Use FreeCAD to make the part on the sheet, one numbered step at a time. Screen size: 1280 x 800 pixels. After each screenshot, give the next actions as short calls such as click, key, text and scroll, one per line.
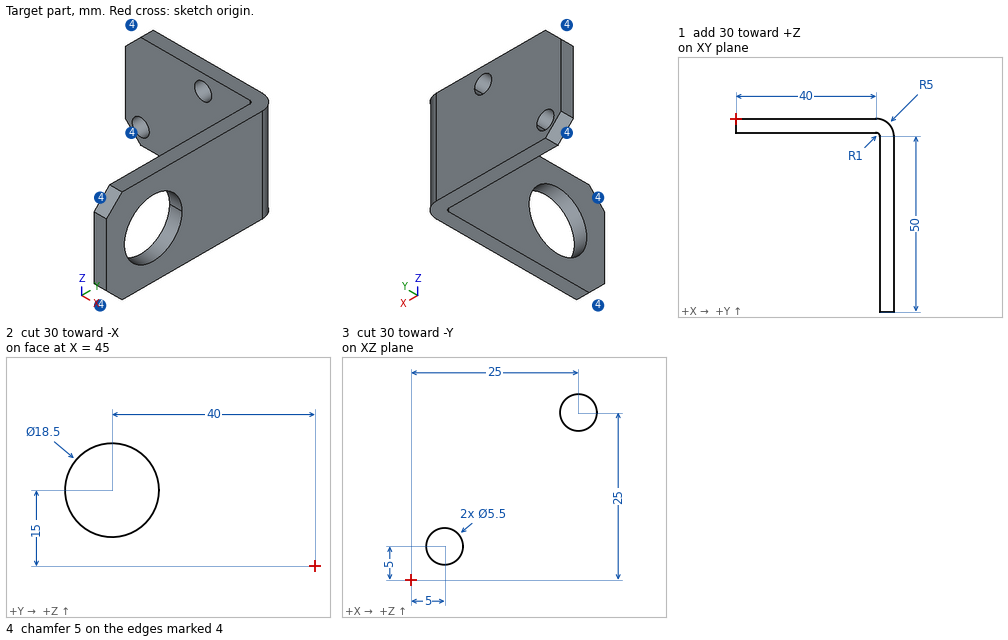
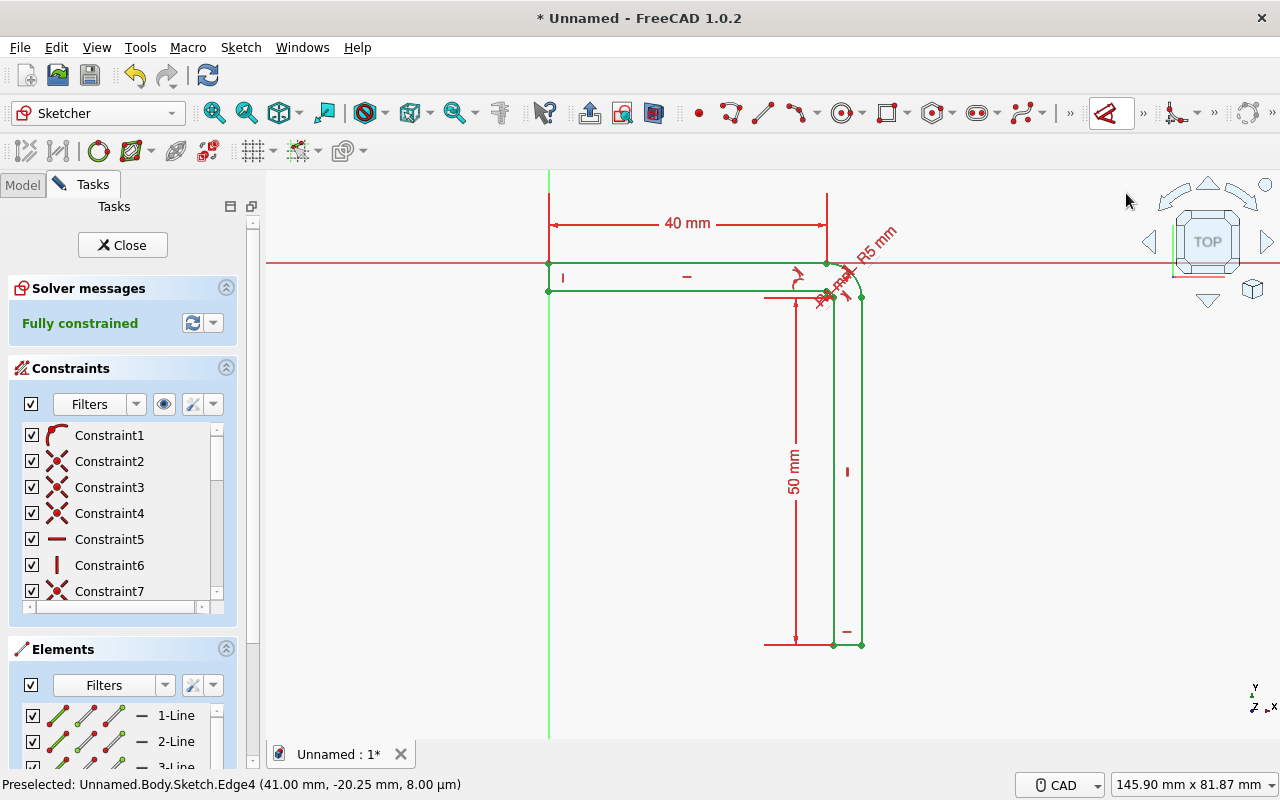
click(123, 245)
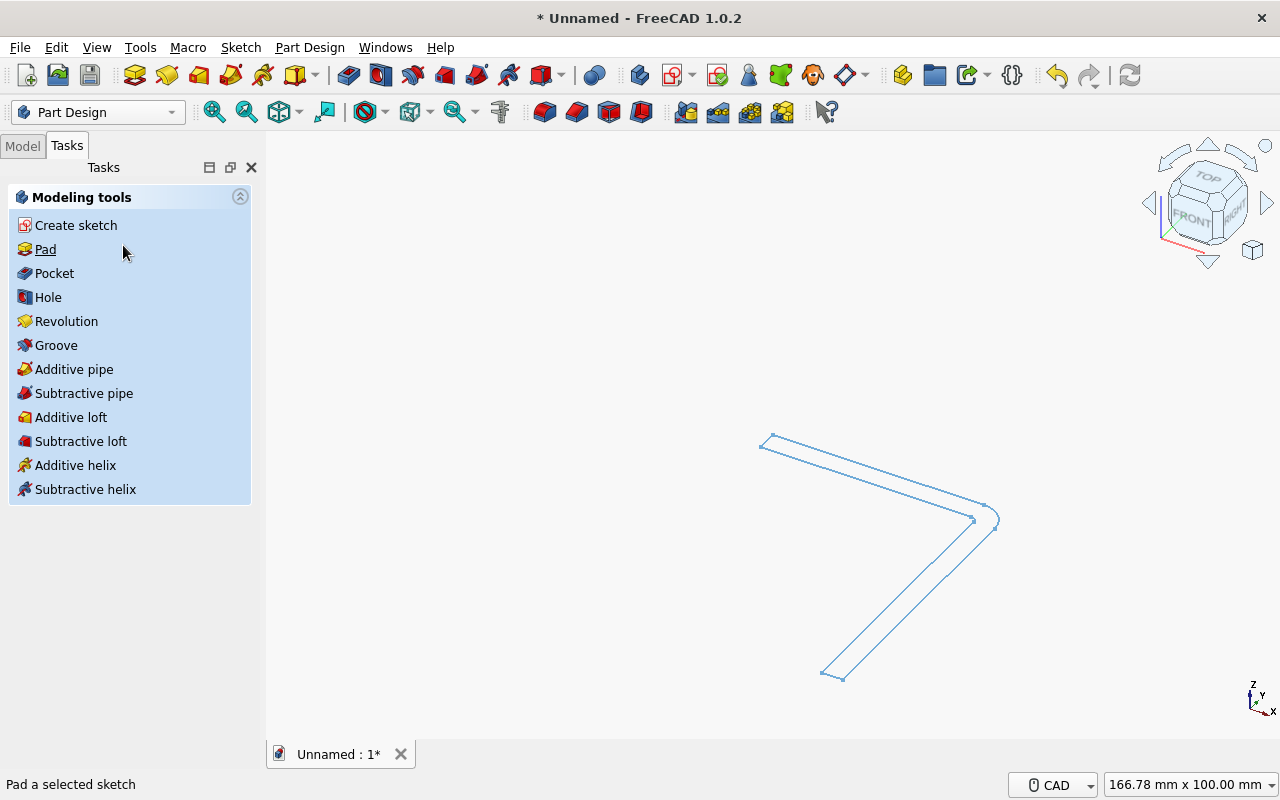
click(136, 76)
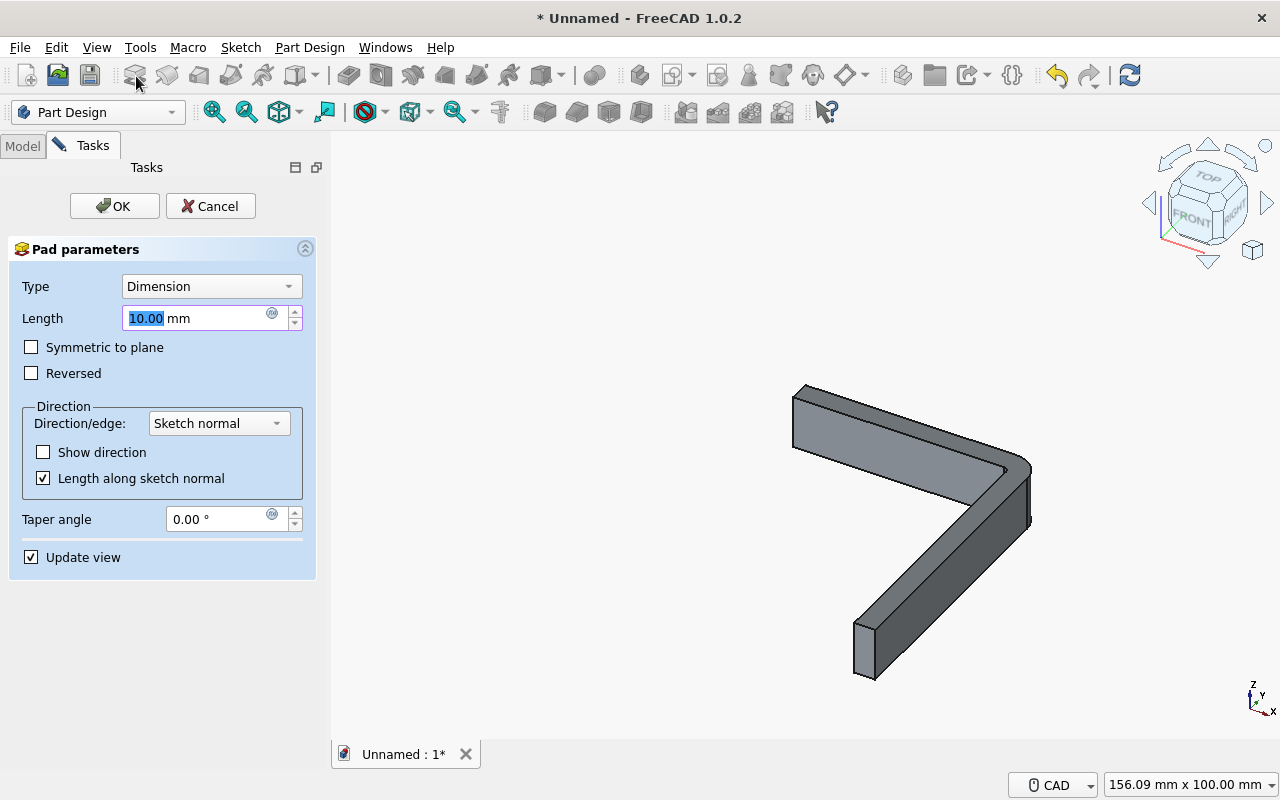
text(30)
key(Tab)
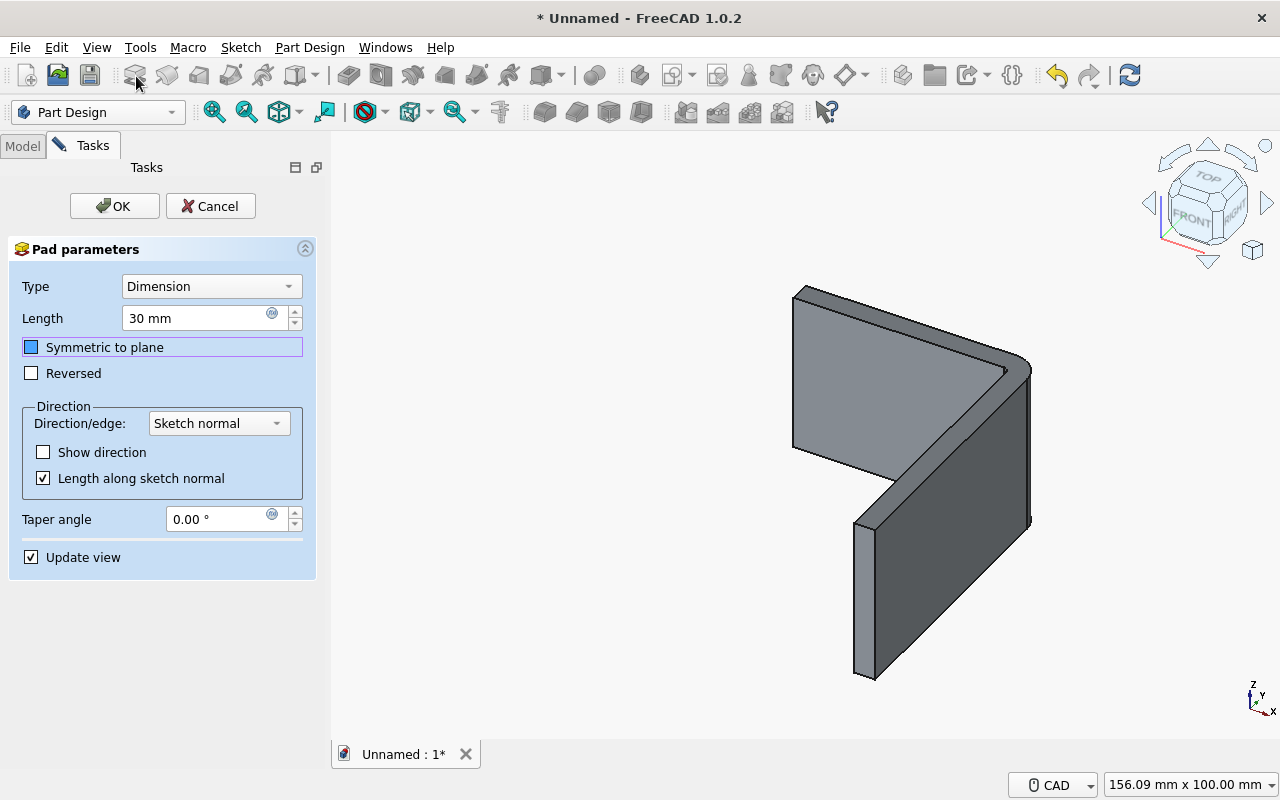
click(115, 206)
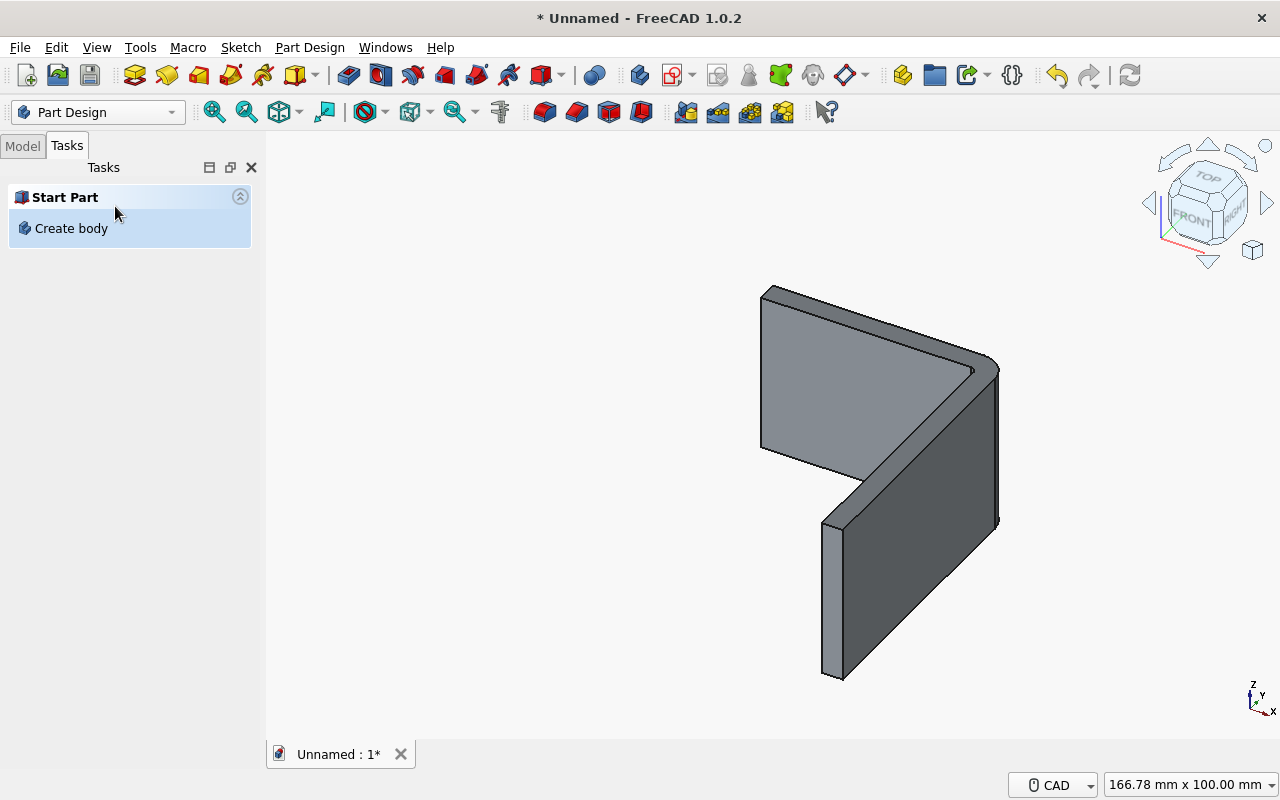
click(940, 507)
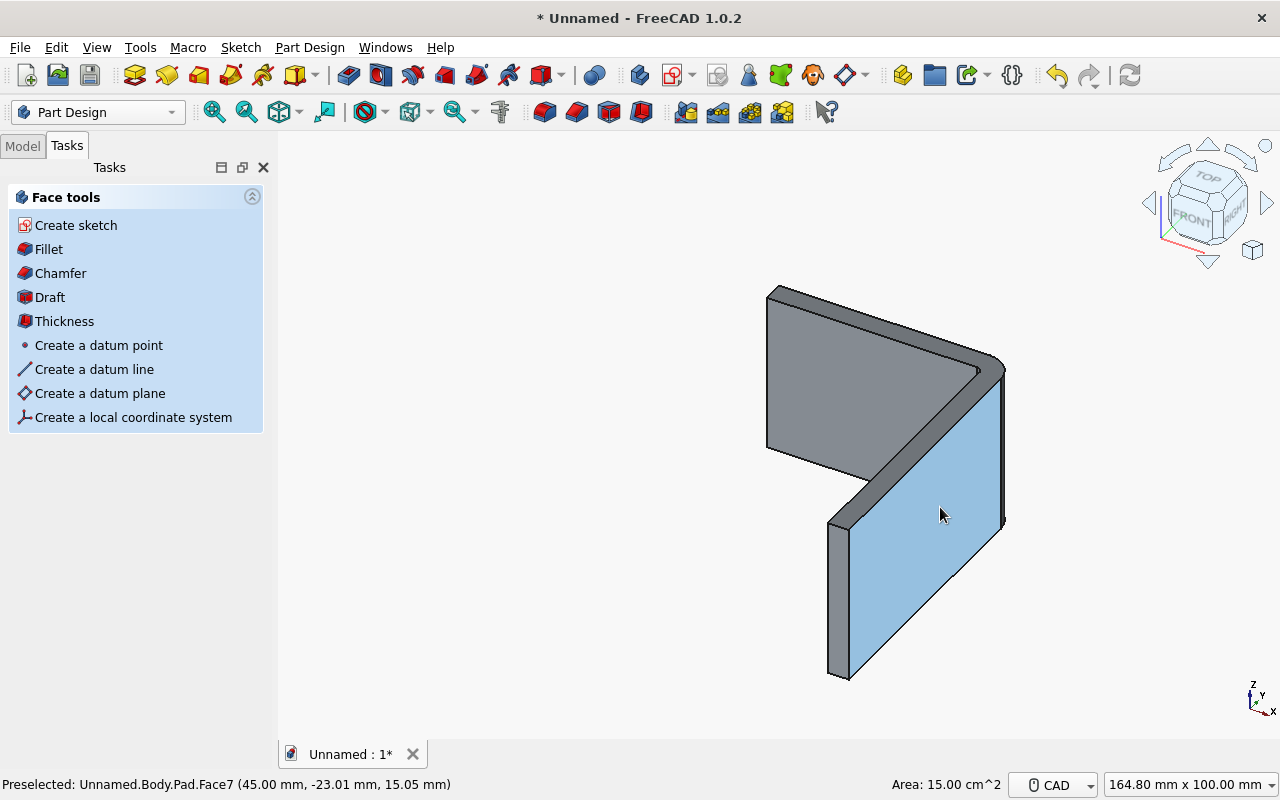
click(672, 76)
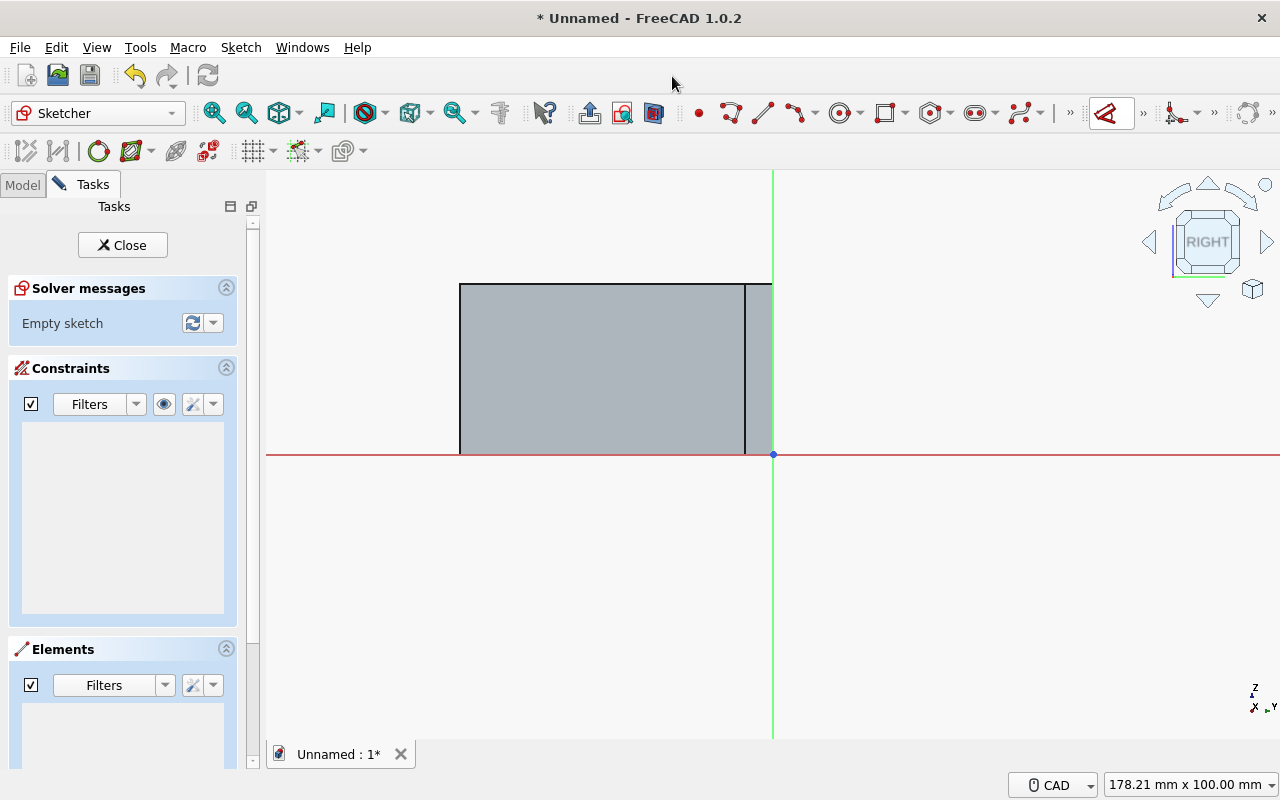
scroll(477, 332, up, 6)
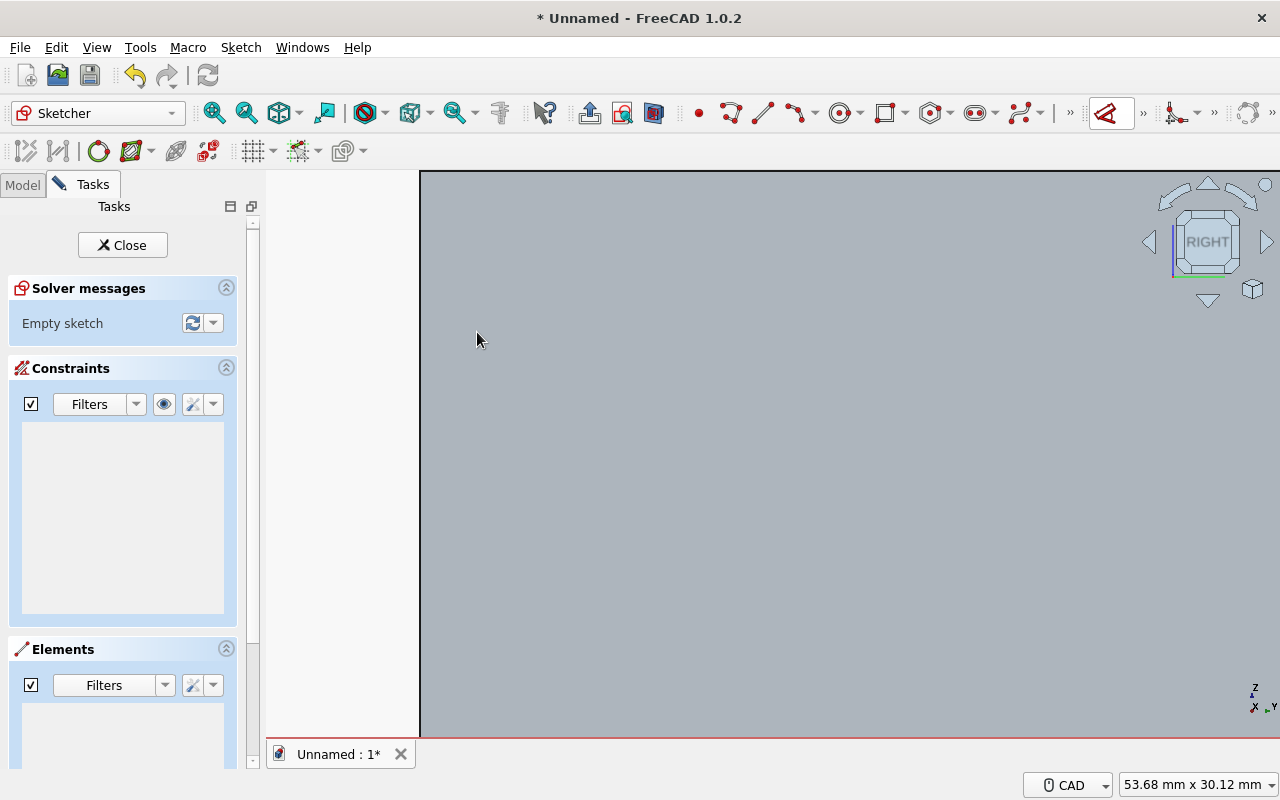
click(840, 114)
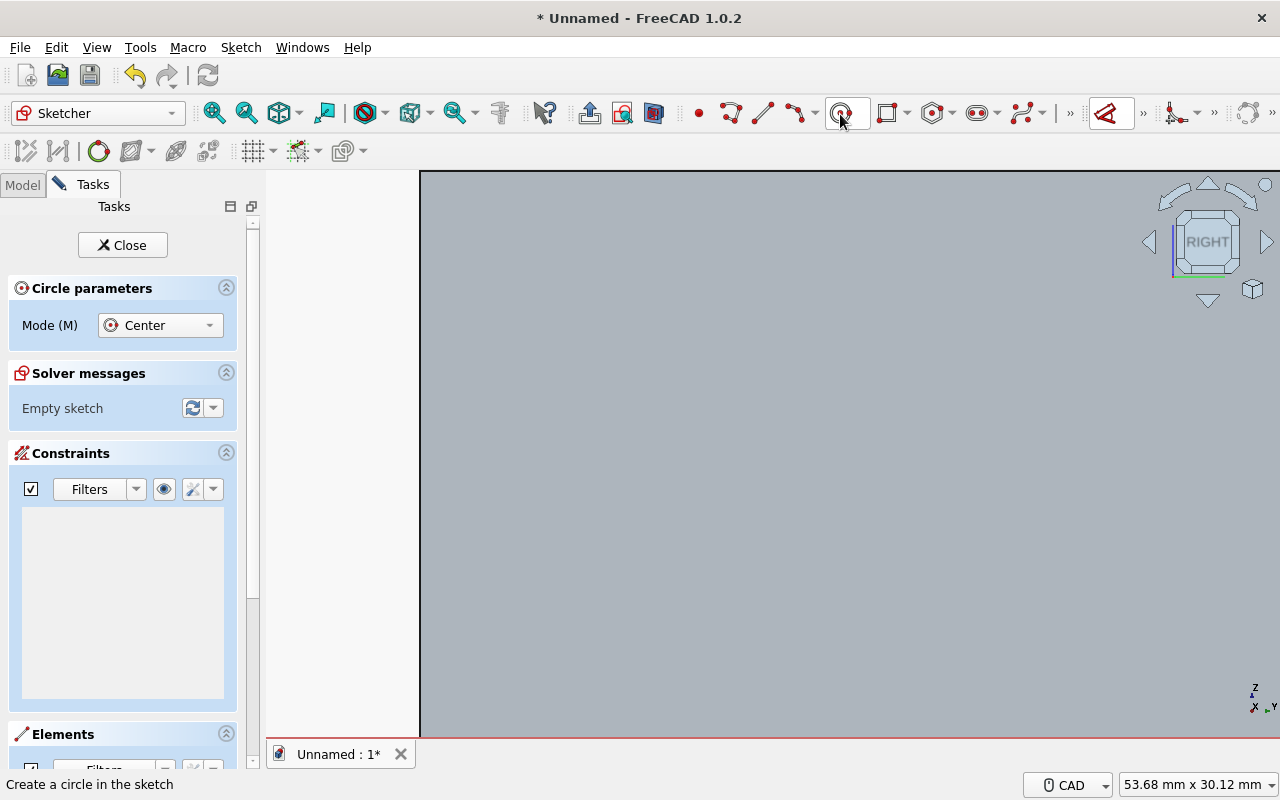
click(704, 455)
click(827, 331)
key(Escape)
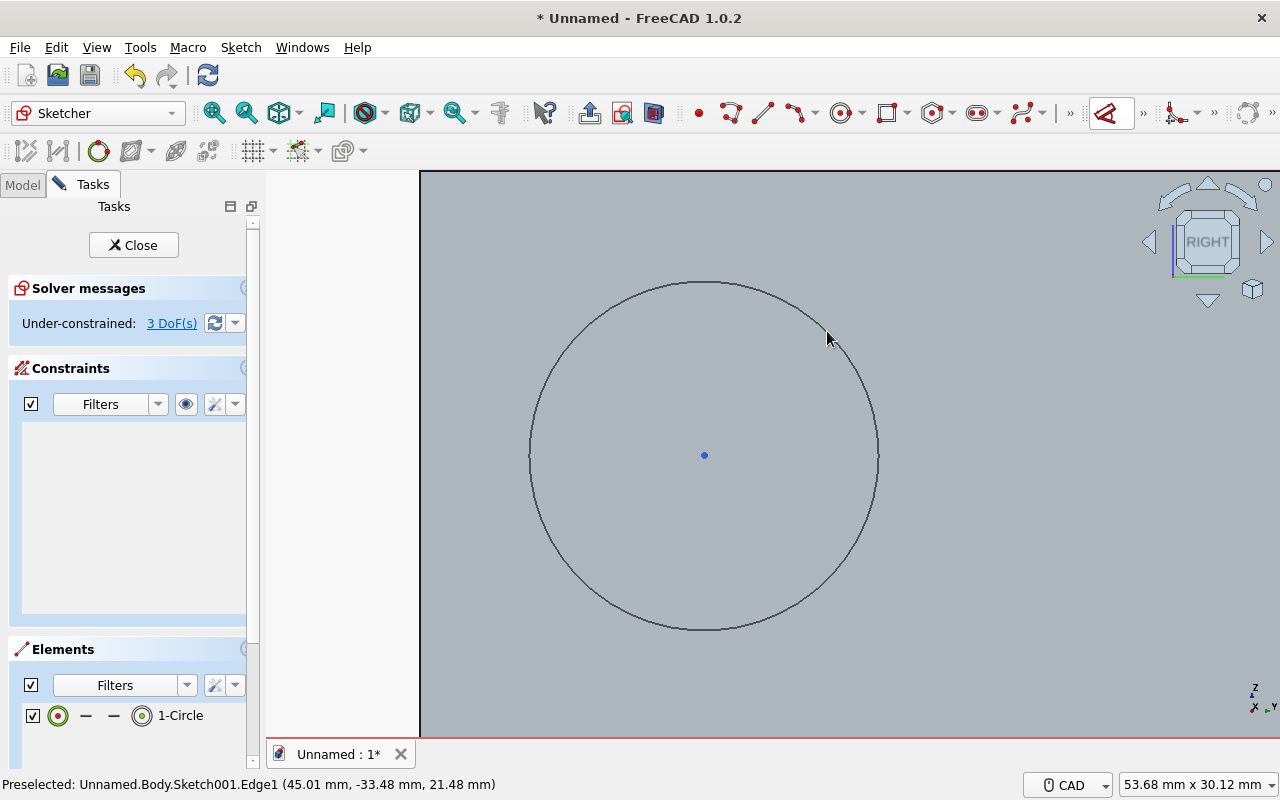
click(827, 332)